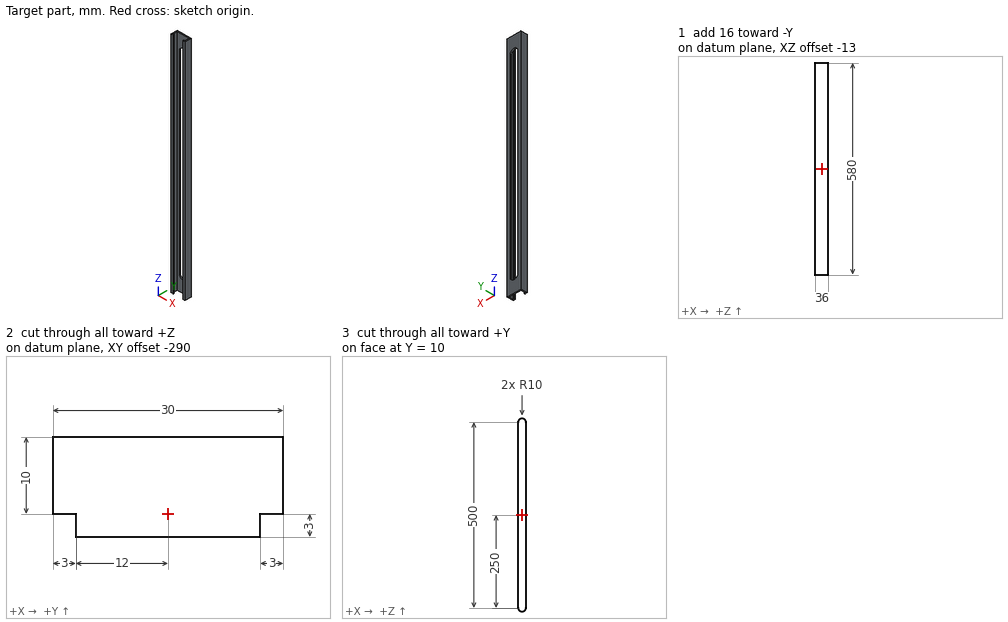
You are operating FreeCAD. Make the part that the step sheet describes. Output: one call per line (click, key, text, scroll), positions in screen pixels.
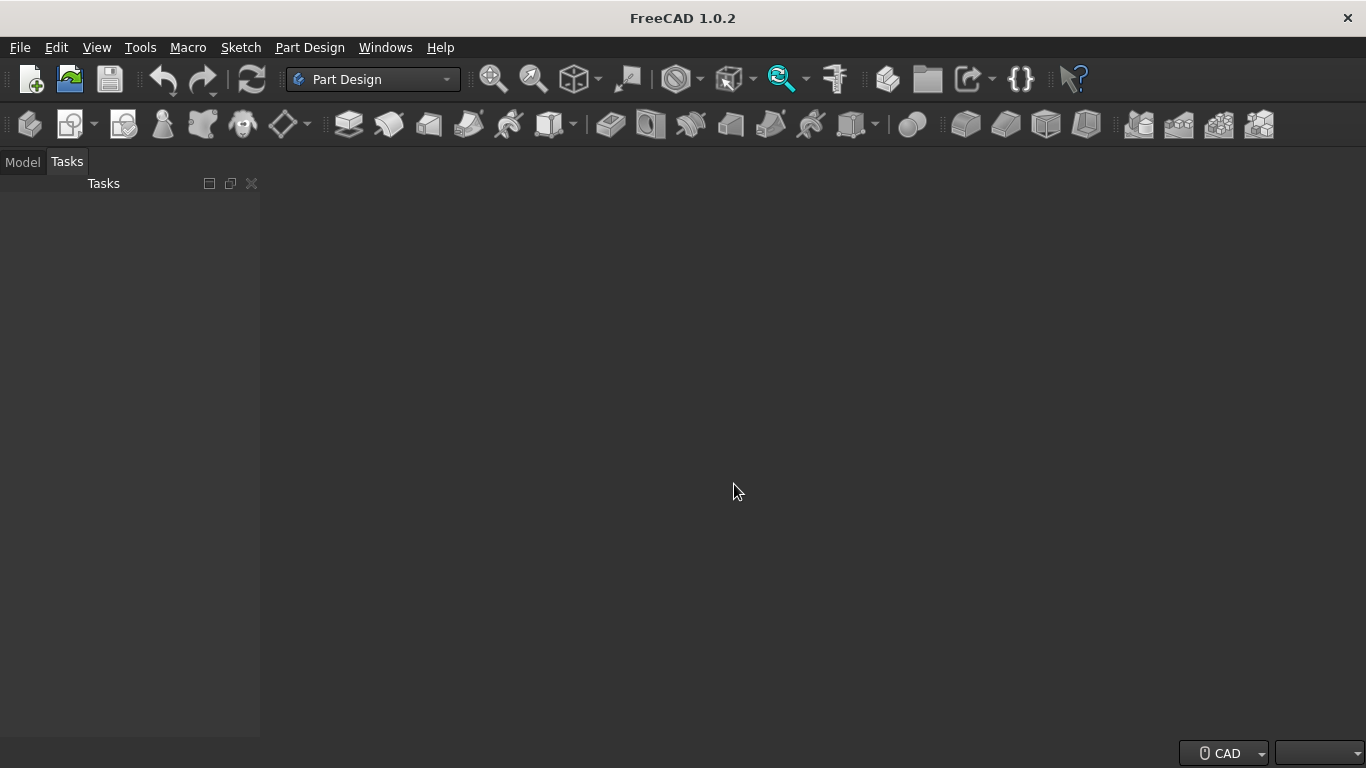
click(30, 80)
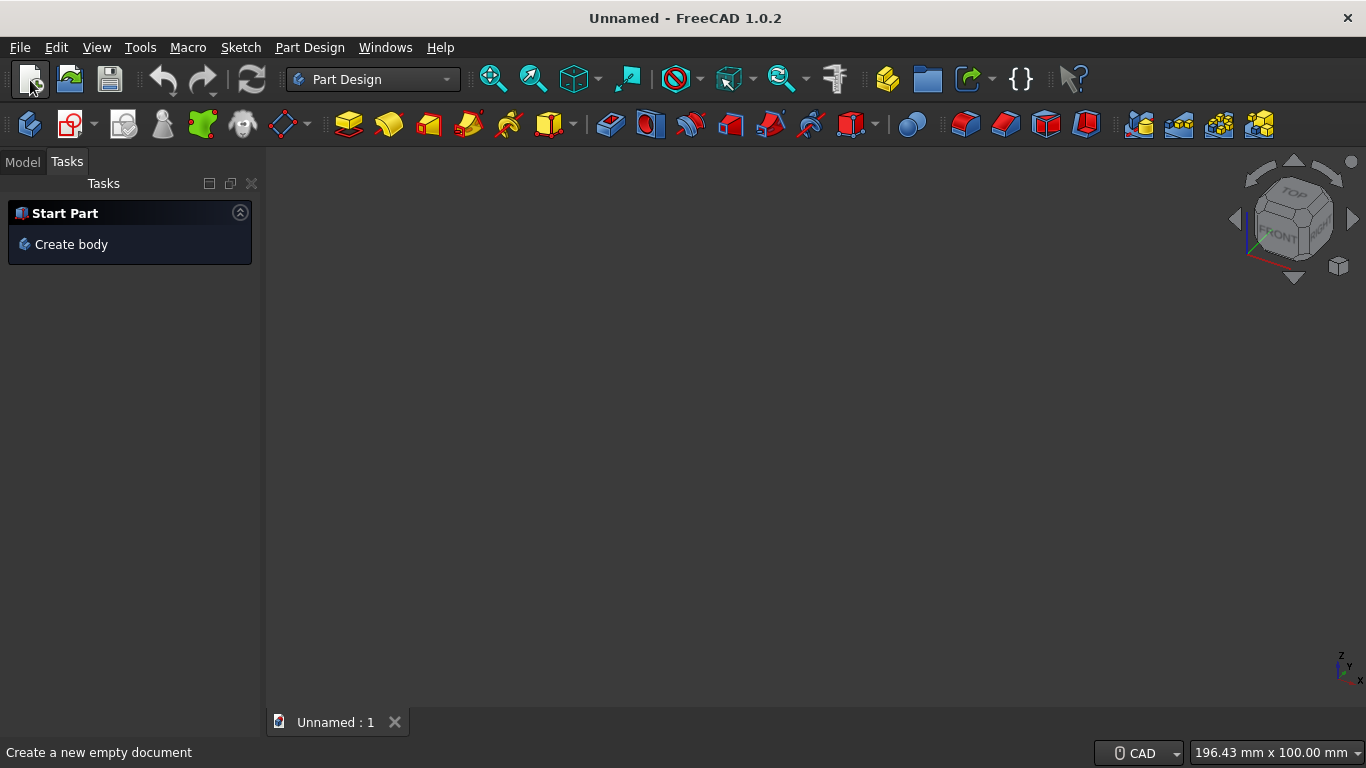
click(30, 124)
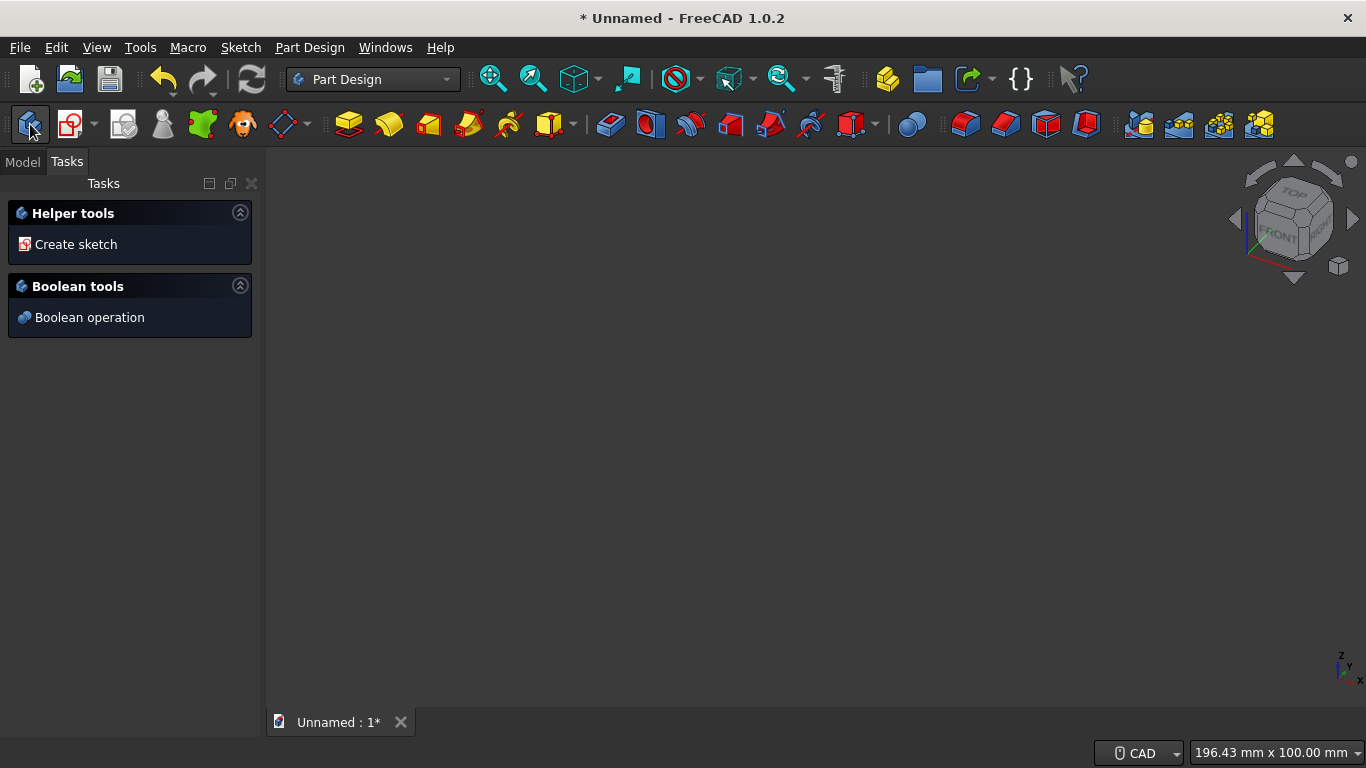
click(23, 161)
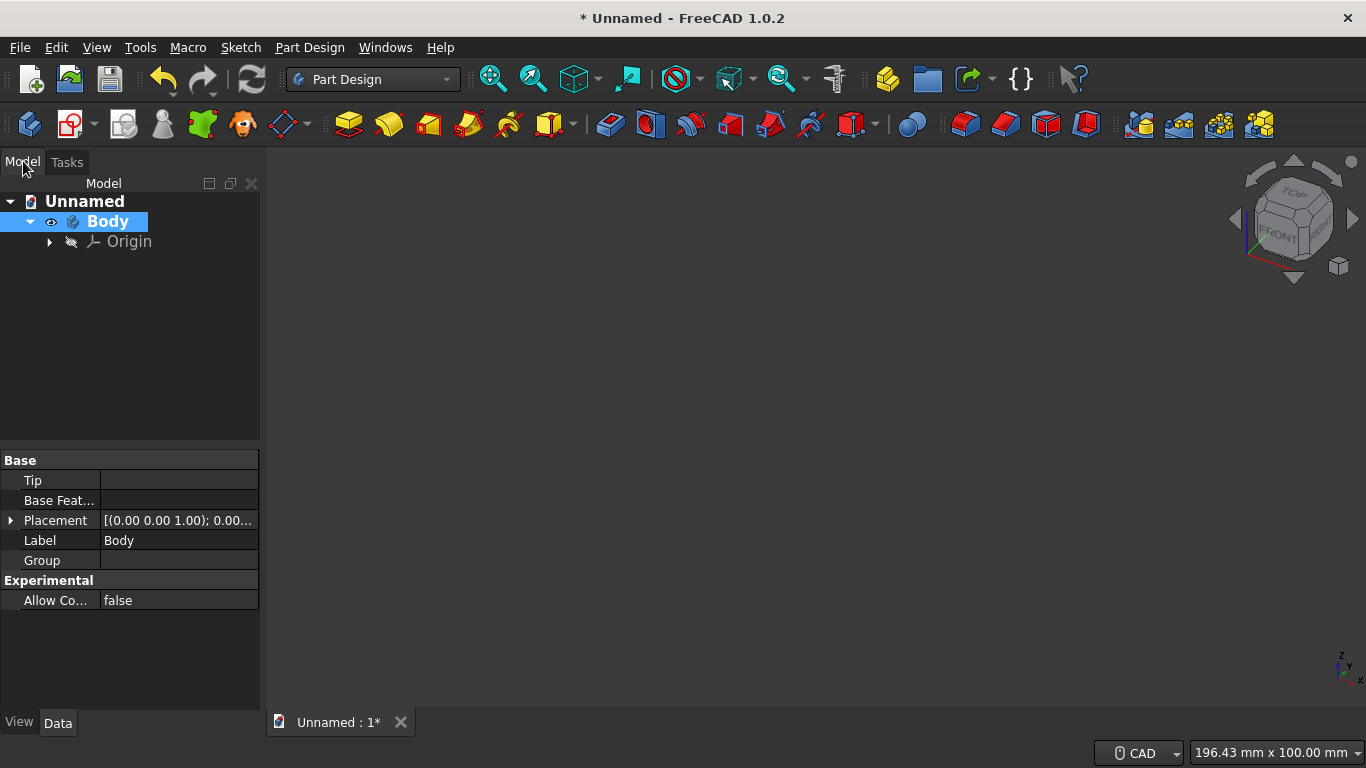
click(50, 242)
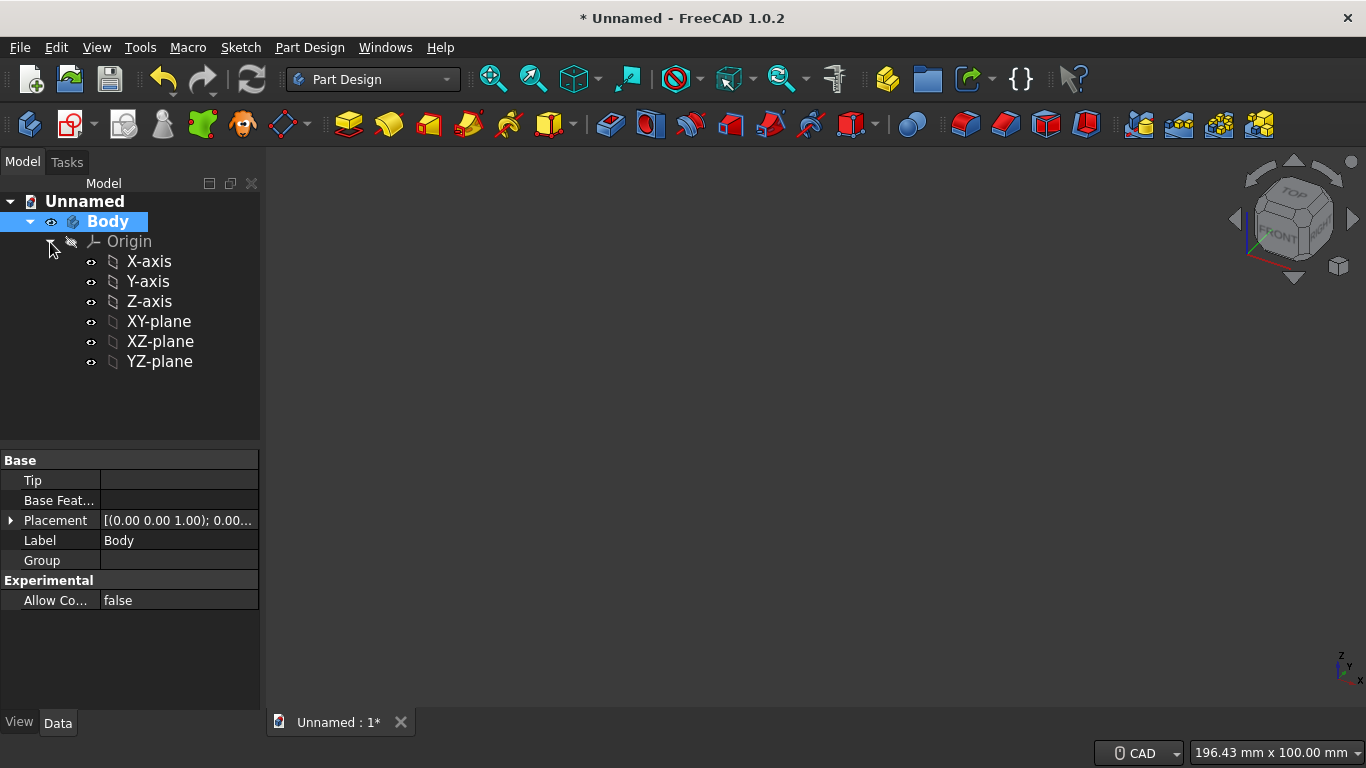
click(136, 342)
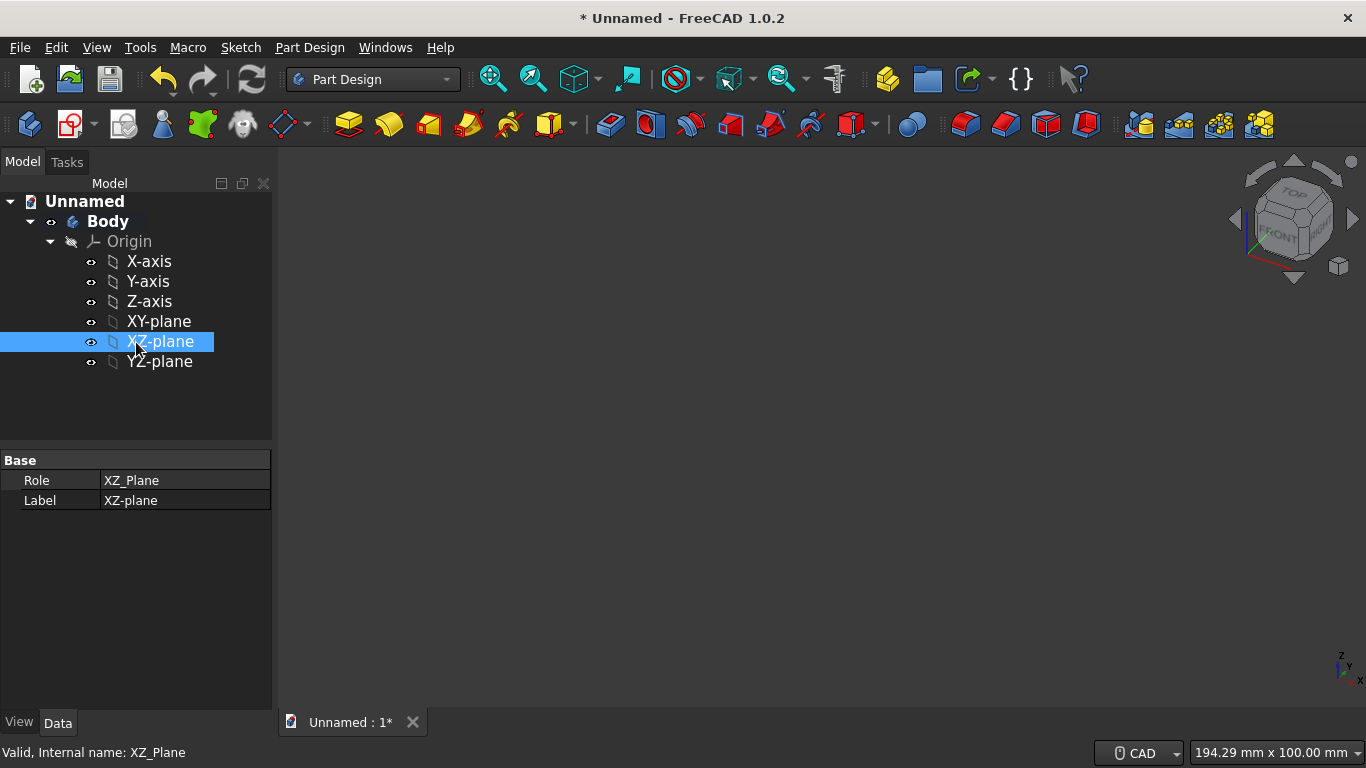
click(284, 124)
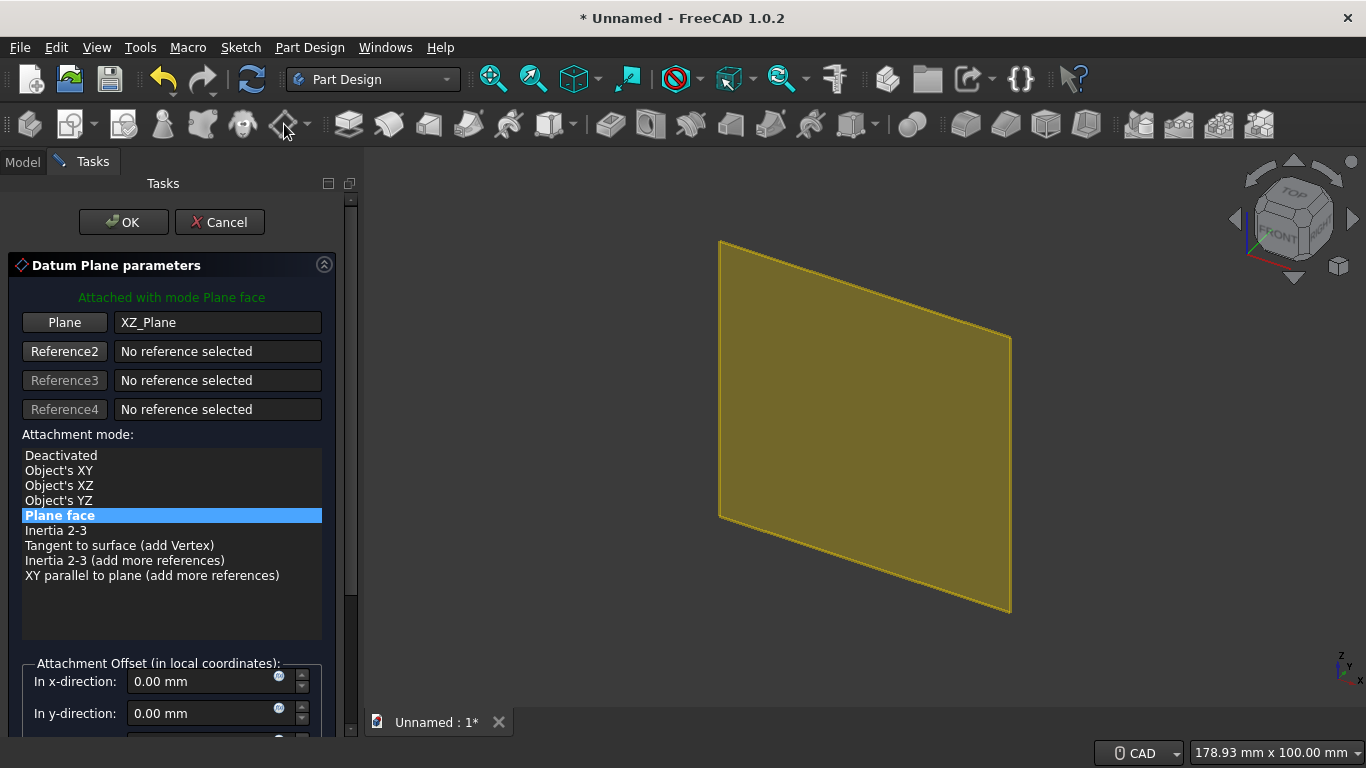
scroll(351, 464, down, 2)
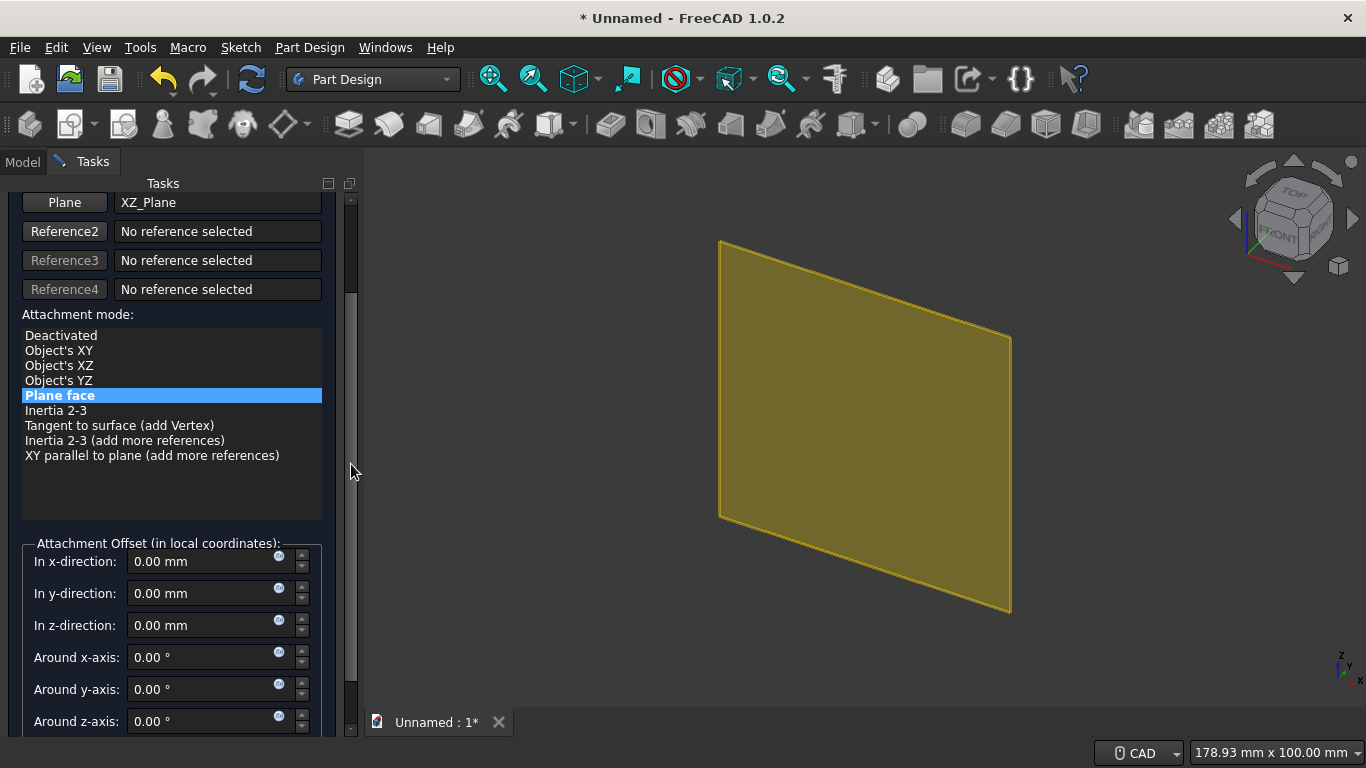
triple_click(210, 625)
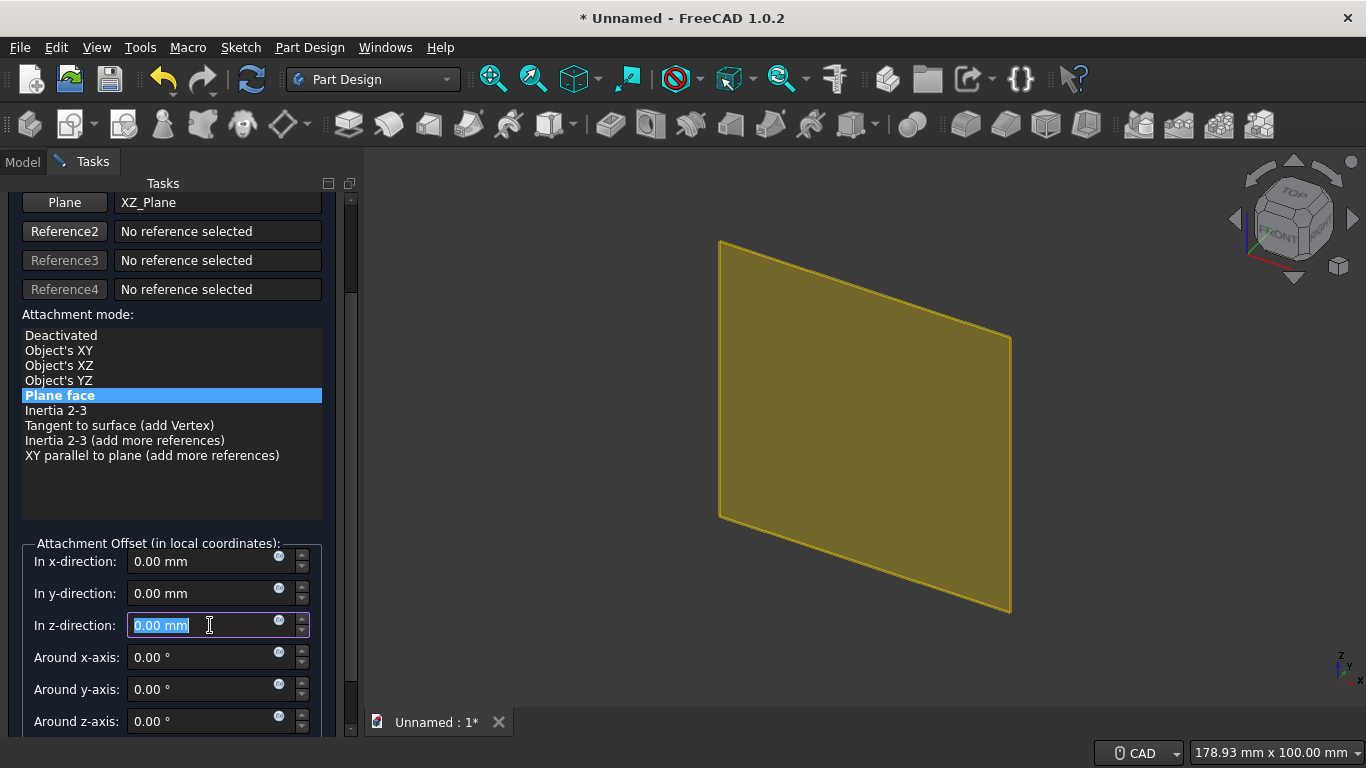
text(-13)
key(Tab)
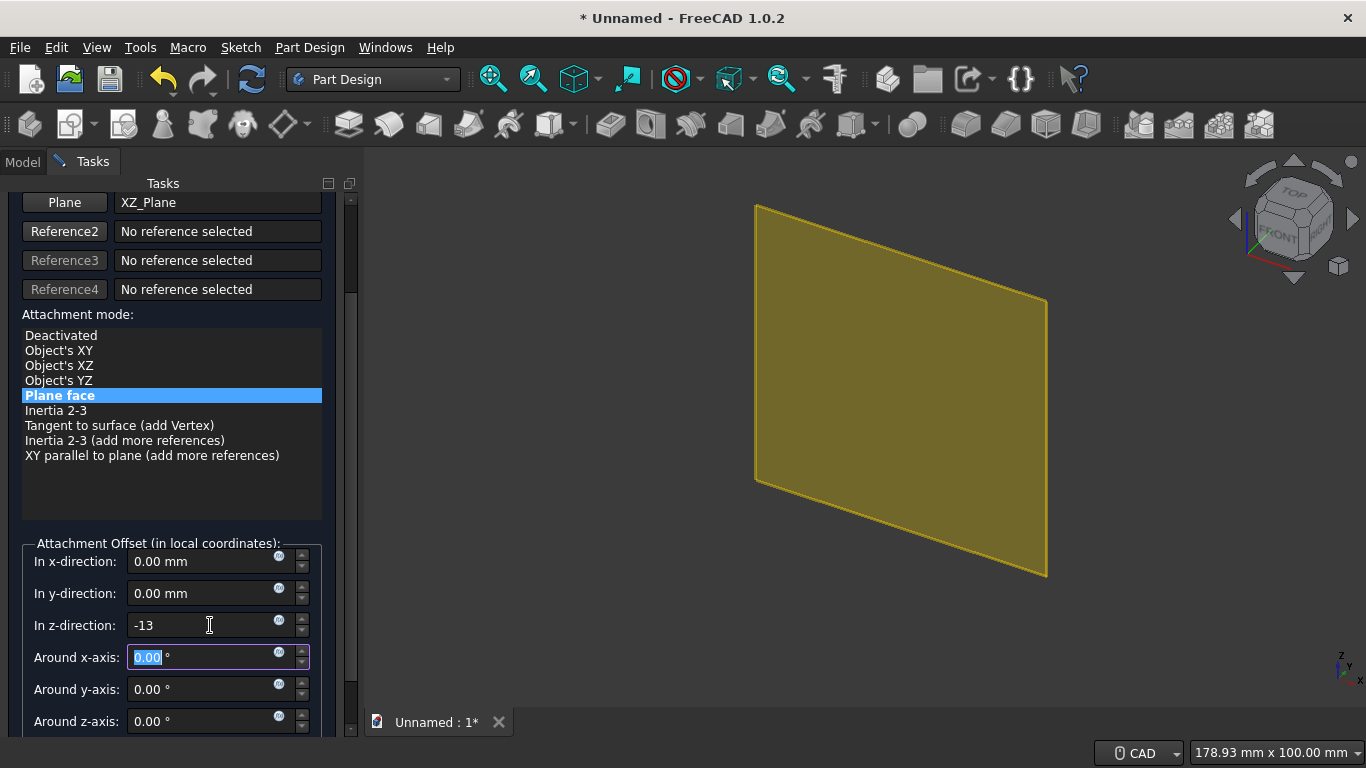
scroll(351, 464, up, 3)